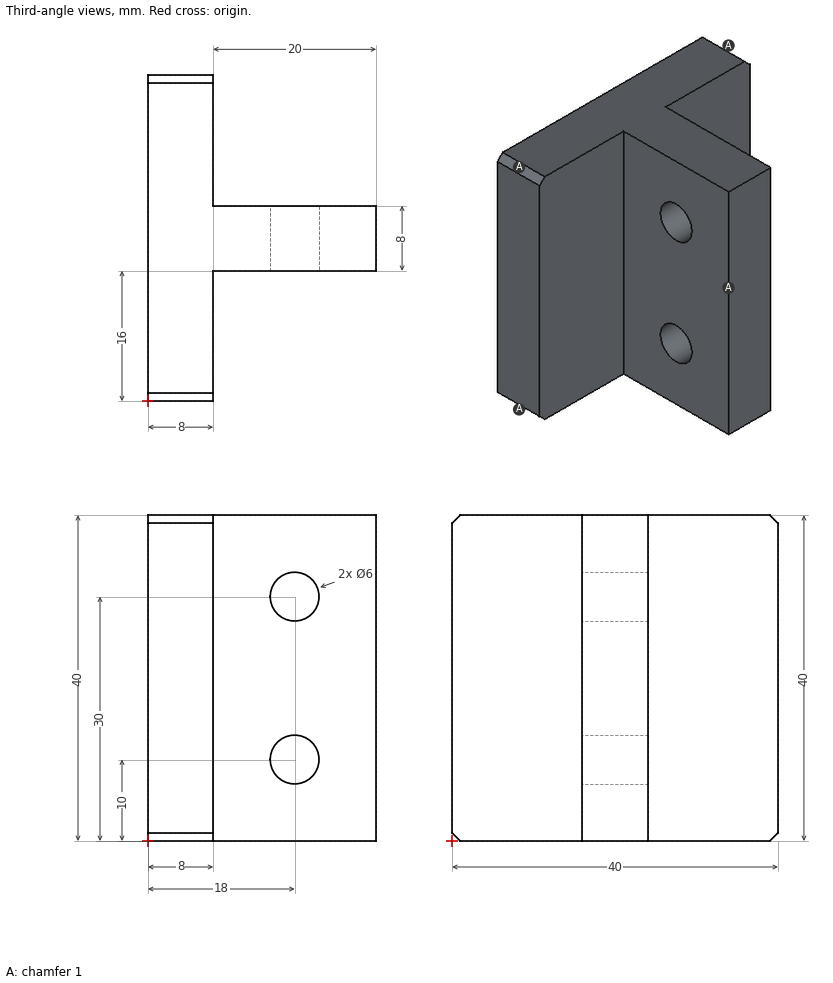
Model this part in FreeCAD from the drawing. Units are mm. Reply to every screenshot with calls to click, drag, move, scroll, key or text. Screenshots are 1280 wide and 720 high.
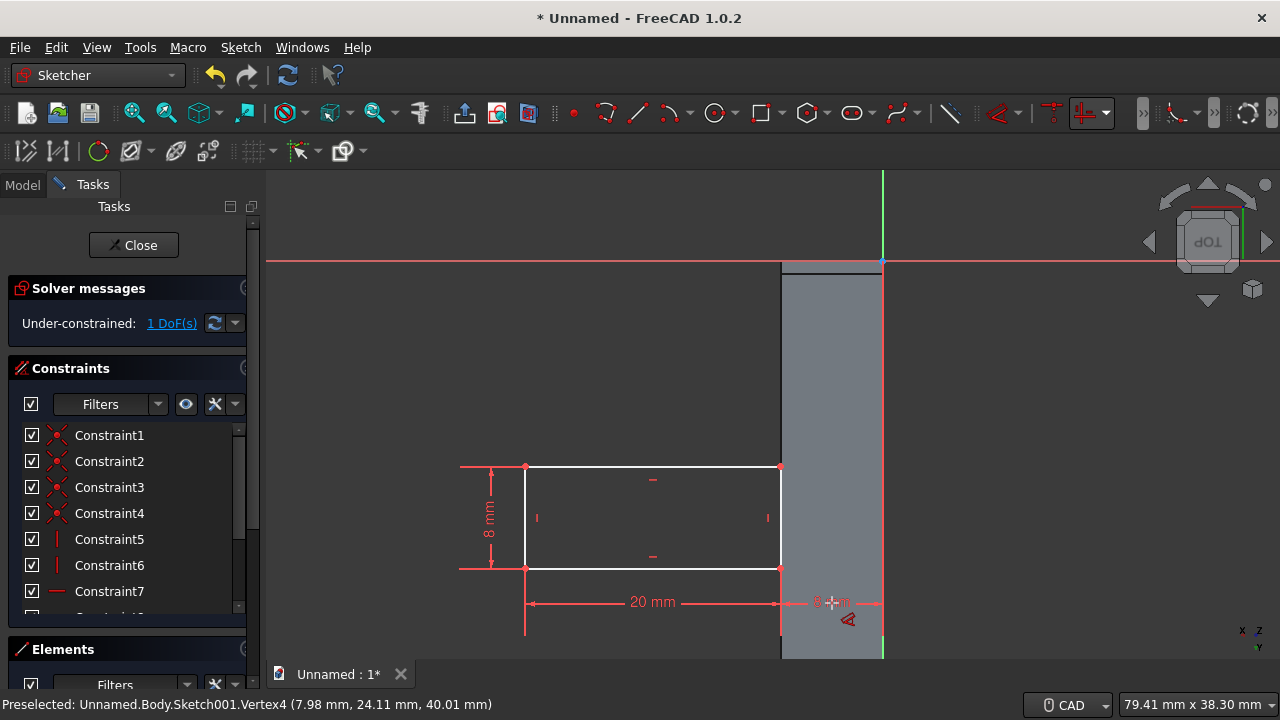
click(525, 467)
click(917, 364)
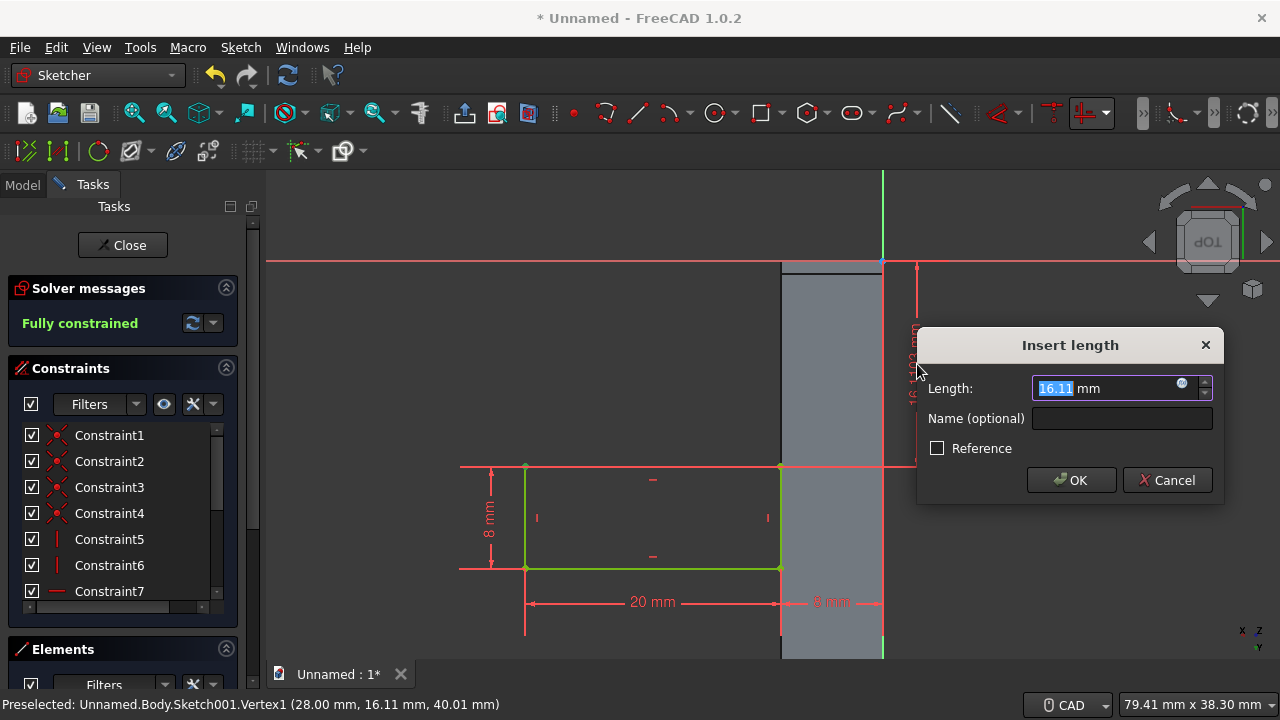
text(16)
key(Return)
key(Escape)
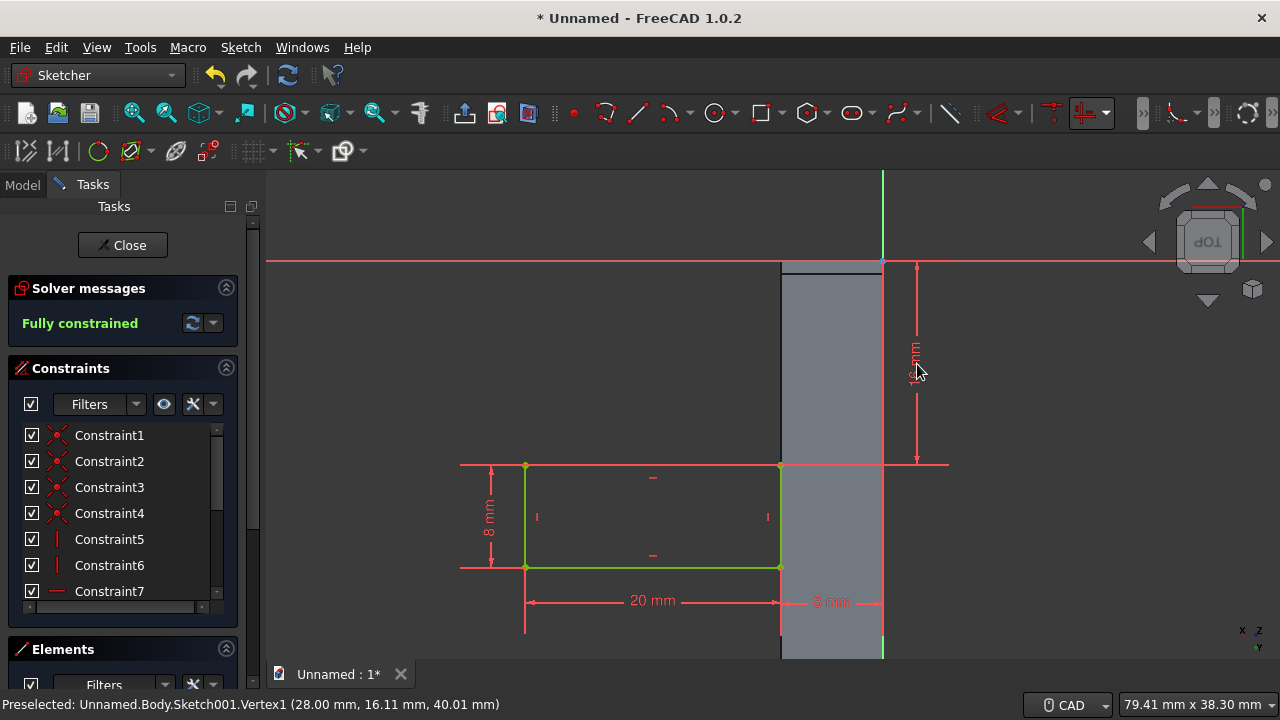
click(123, 245)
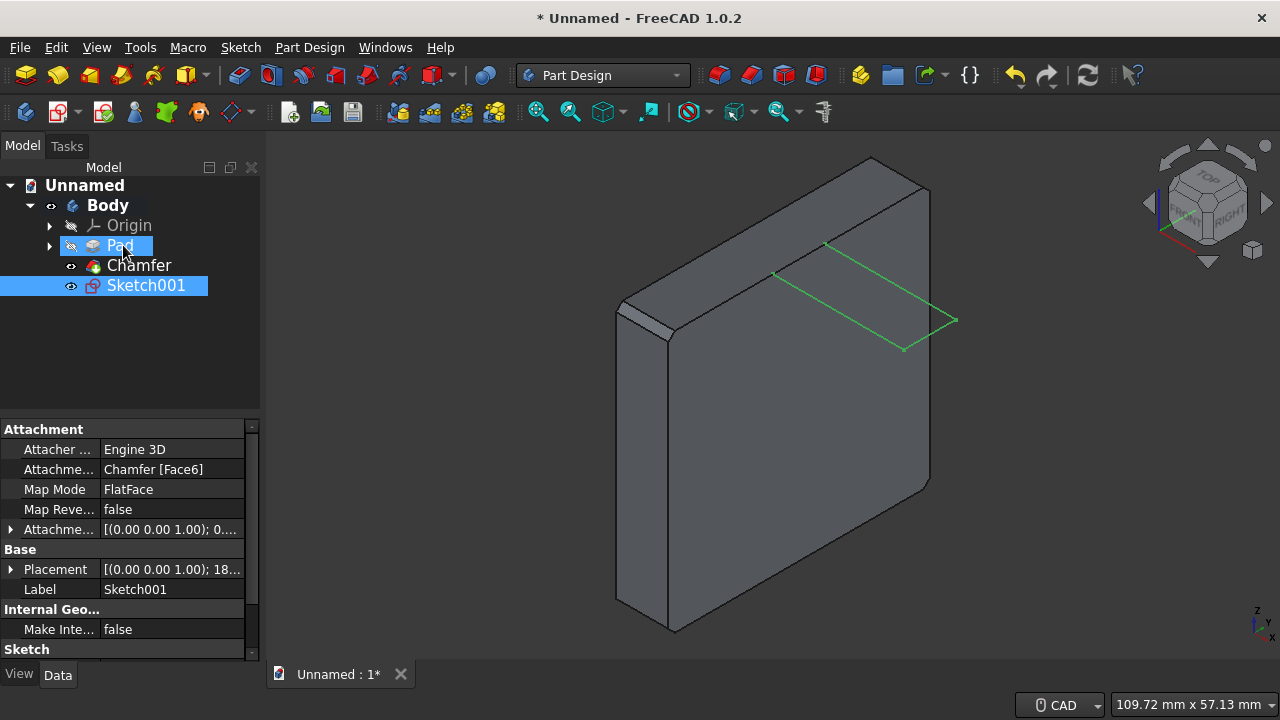
click(26, 76)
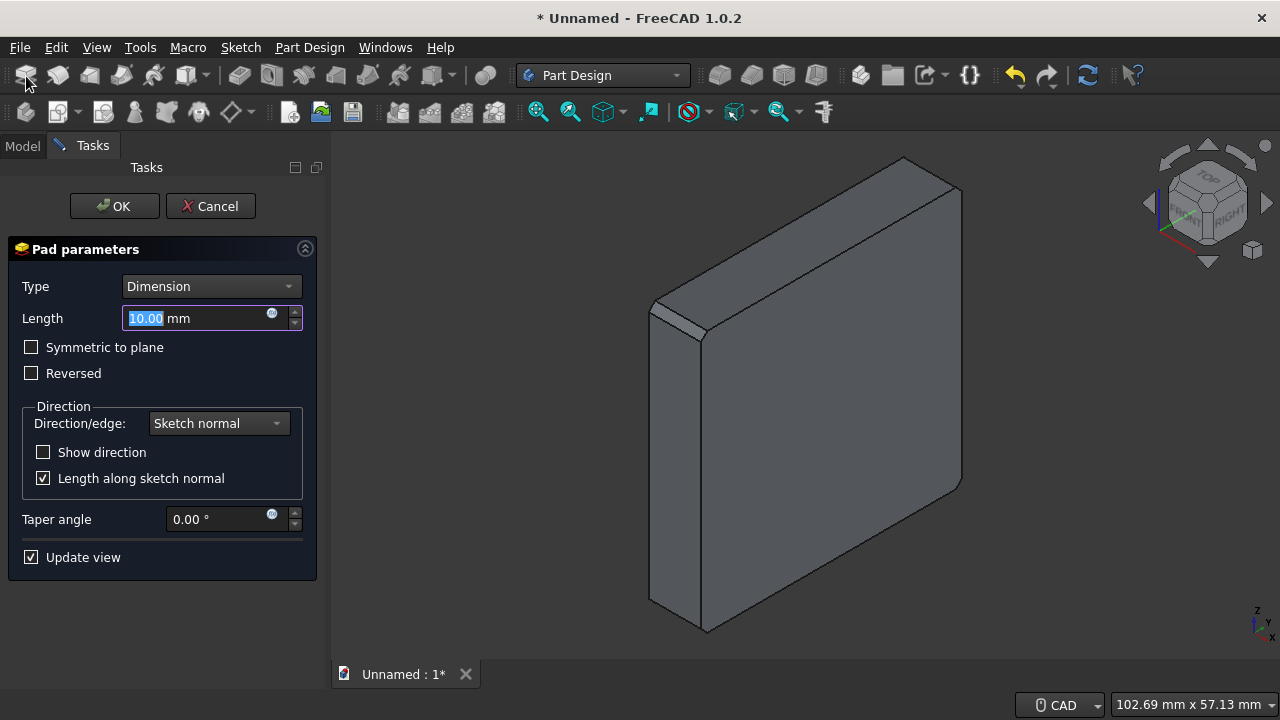
text(40)
key(Tab)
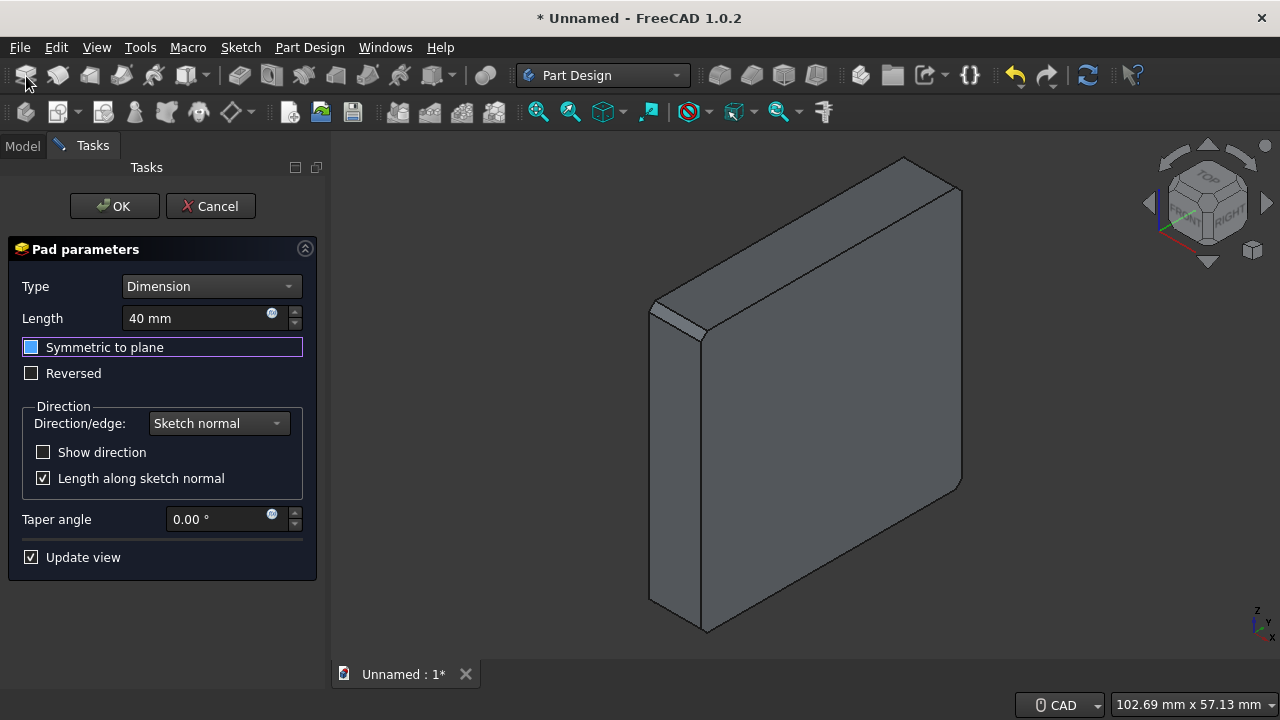
click(30, 373)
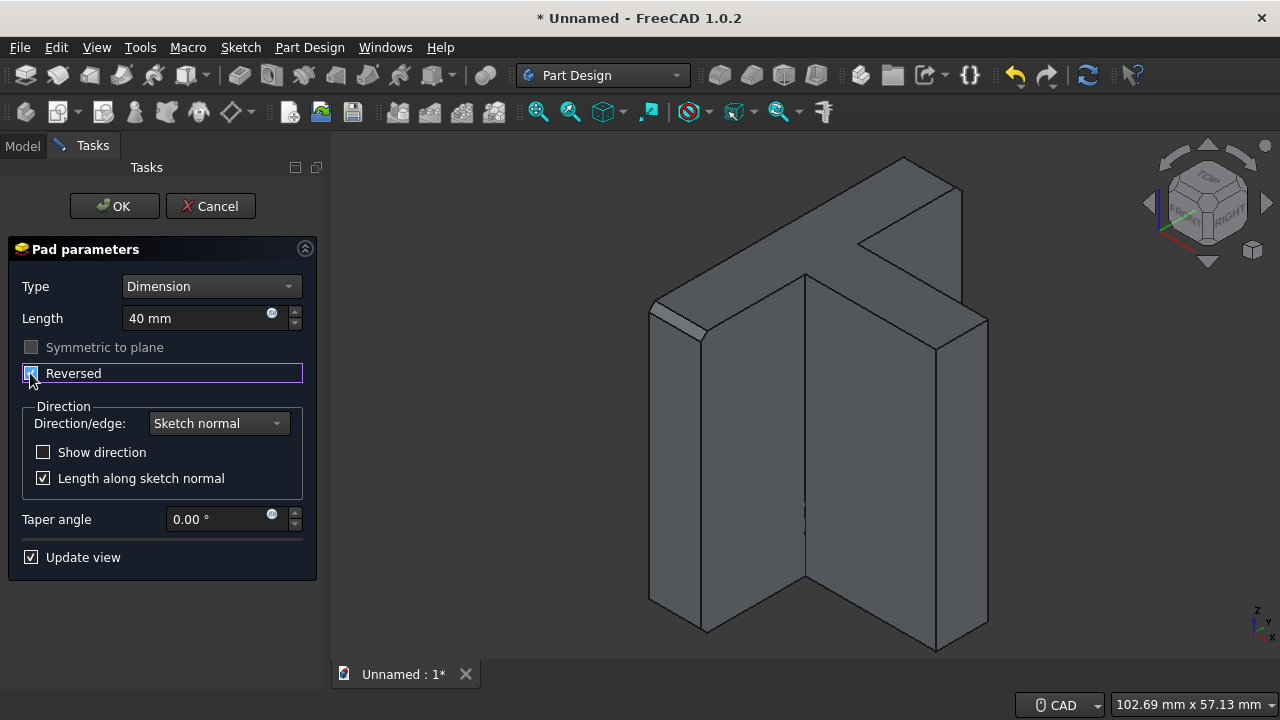
click(115, 206)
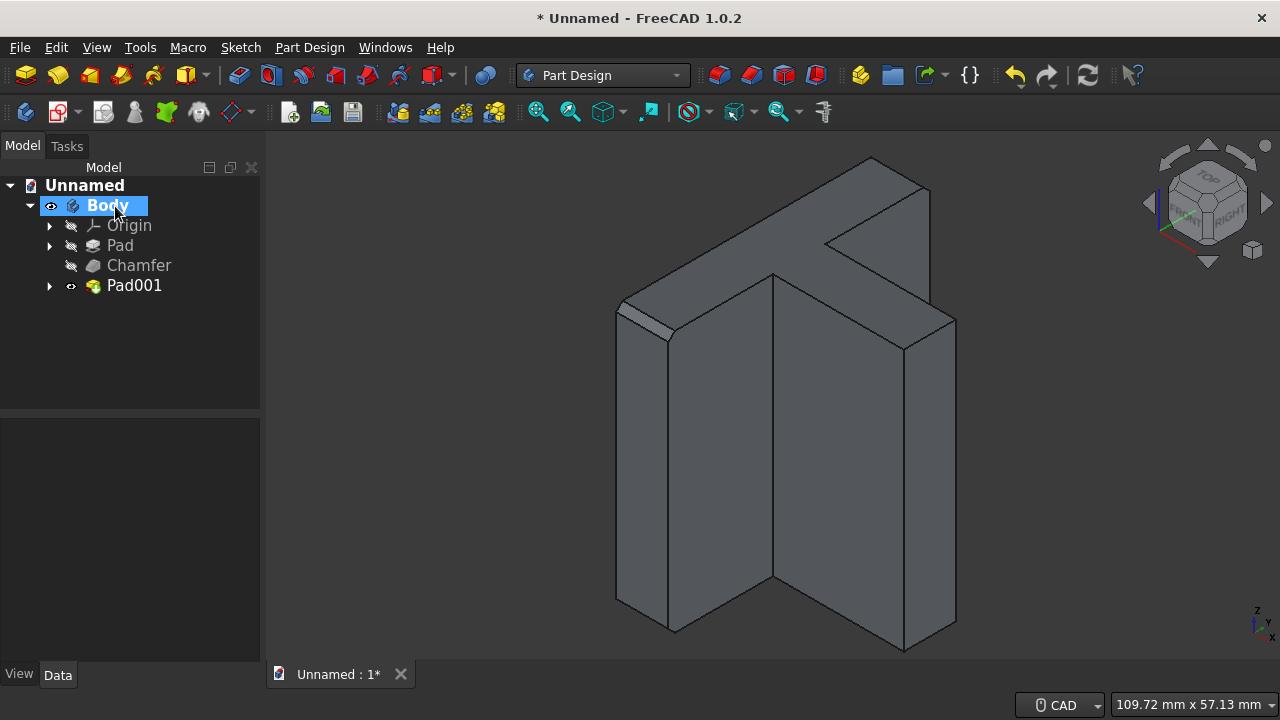
key(v)
key(f)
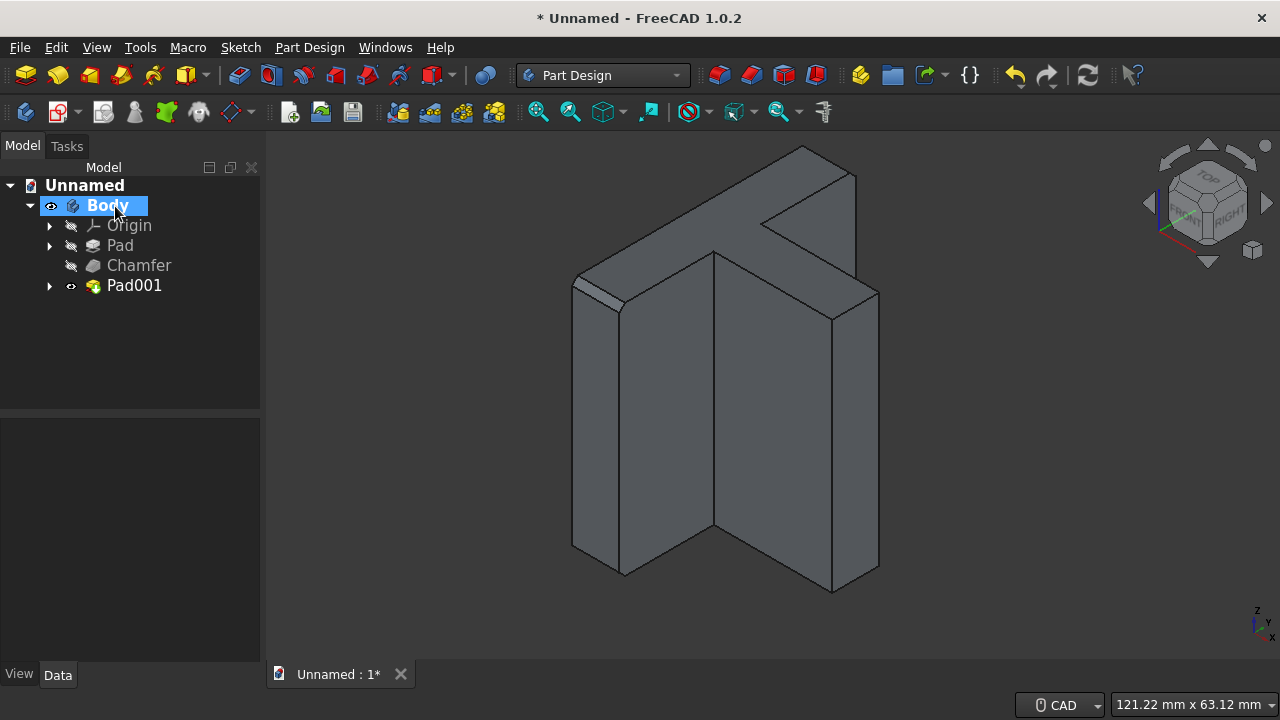
key(4)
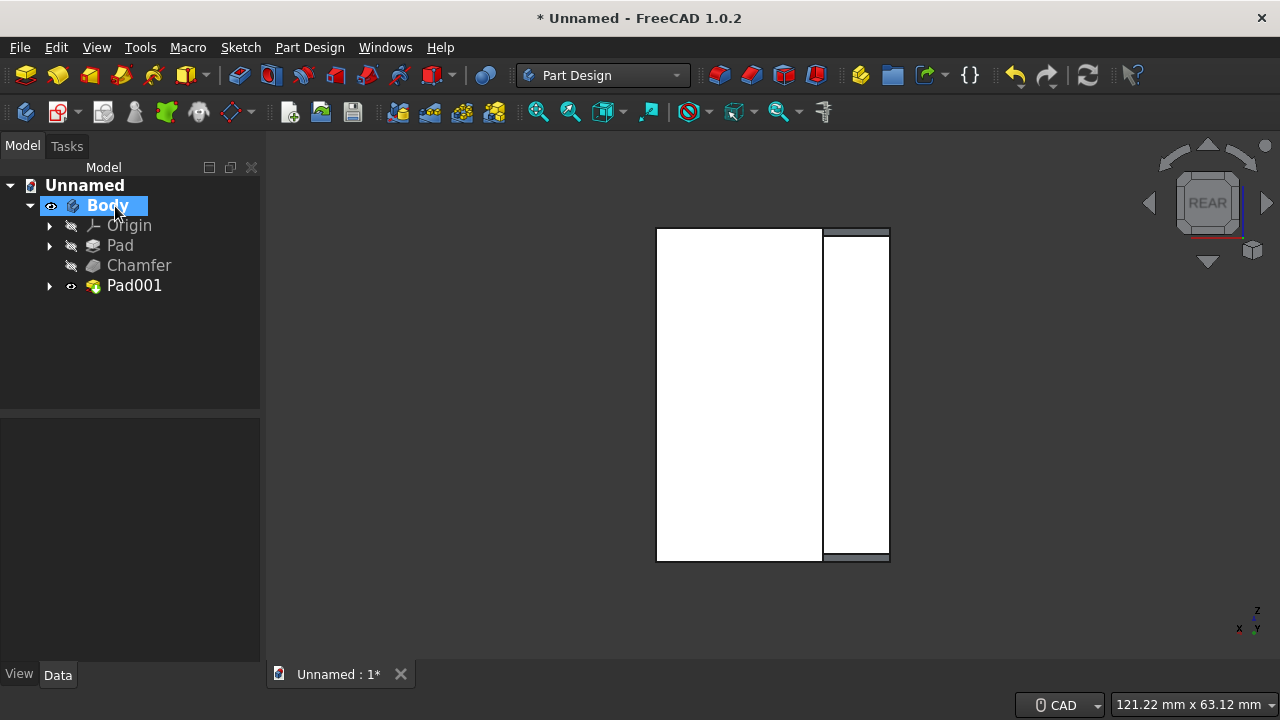
click(740, 394)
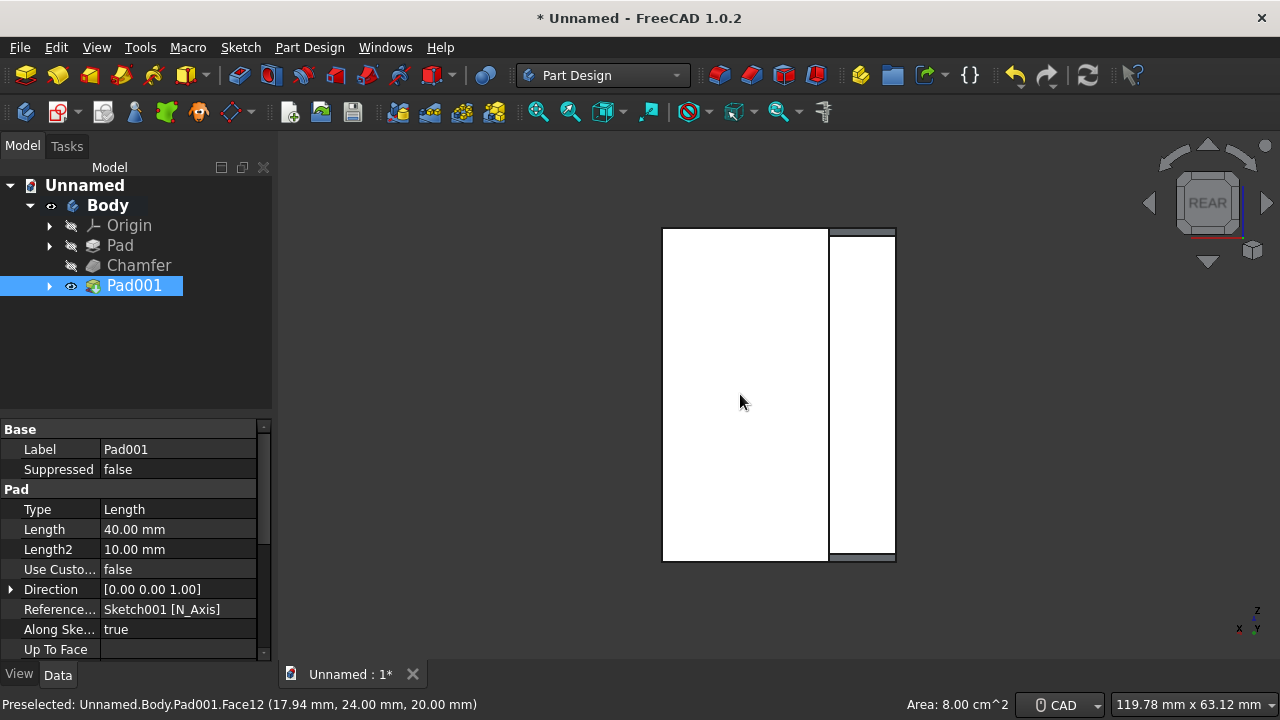
click(58, 112)